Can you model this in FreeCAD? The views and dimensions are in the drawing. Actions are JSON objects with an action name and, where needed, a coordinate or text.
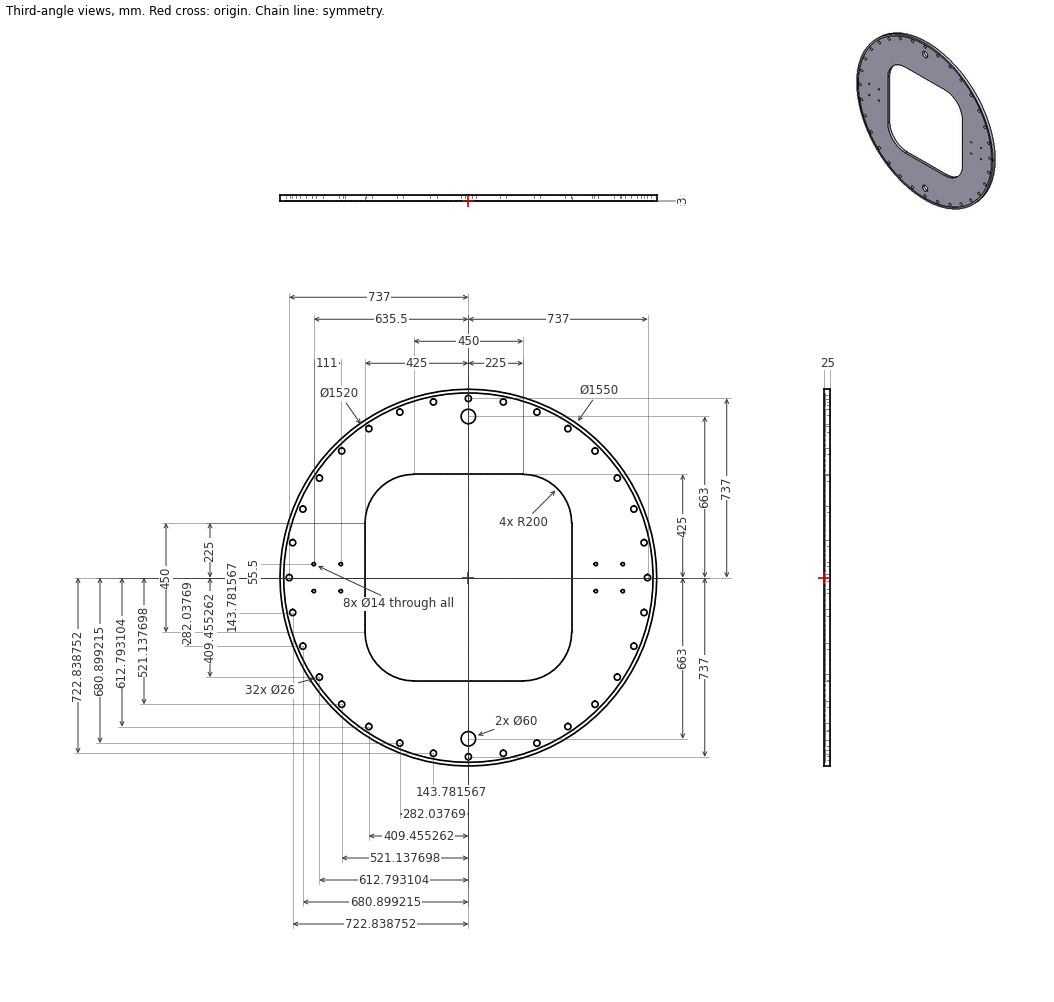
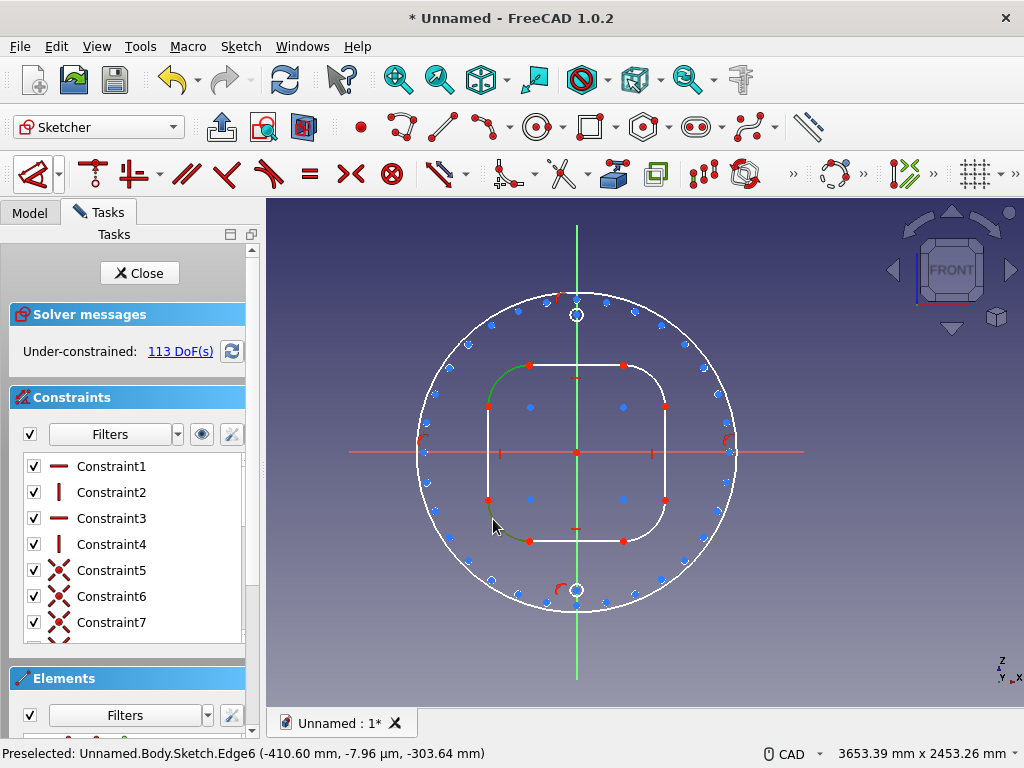
{"action": "left_click", "coordinate": [642, 537]}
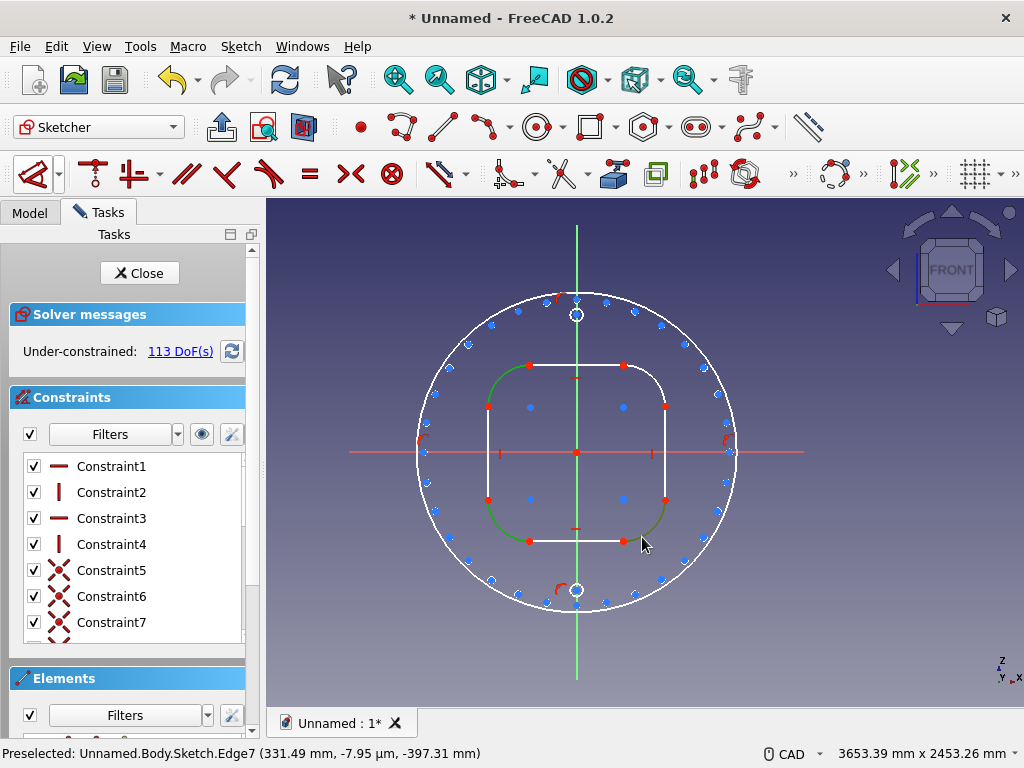
{"action": "left_click", "coordinate": [660, 388]}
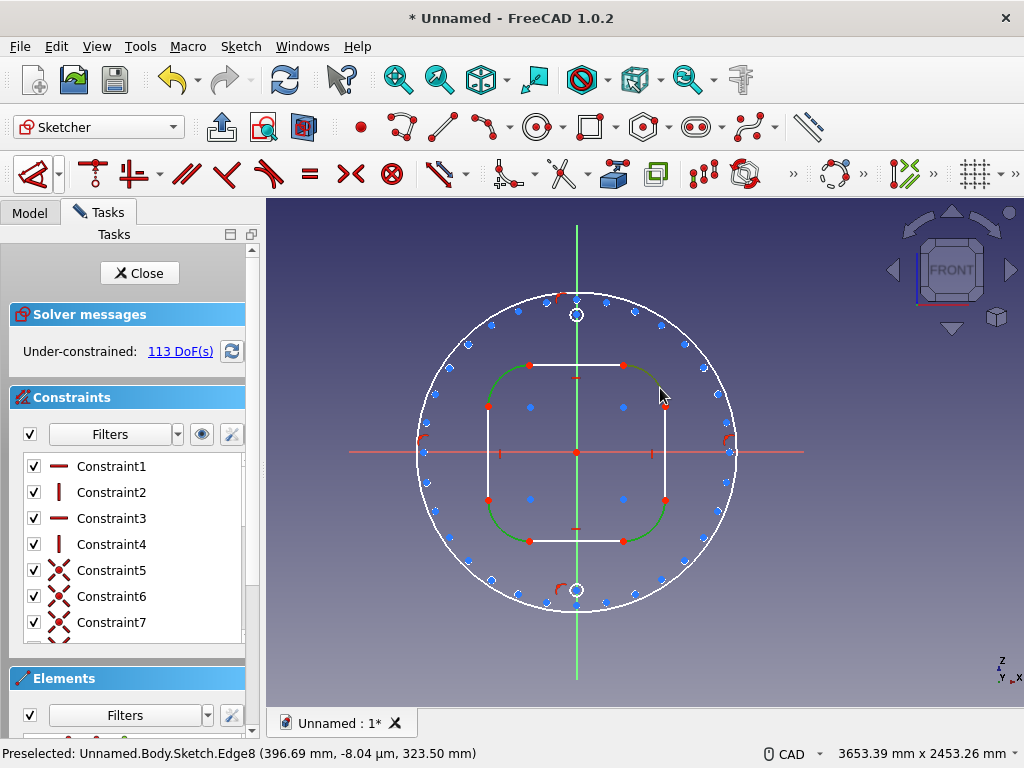
{"action": "left_click", "coordinate": [310, 174]}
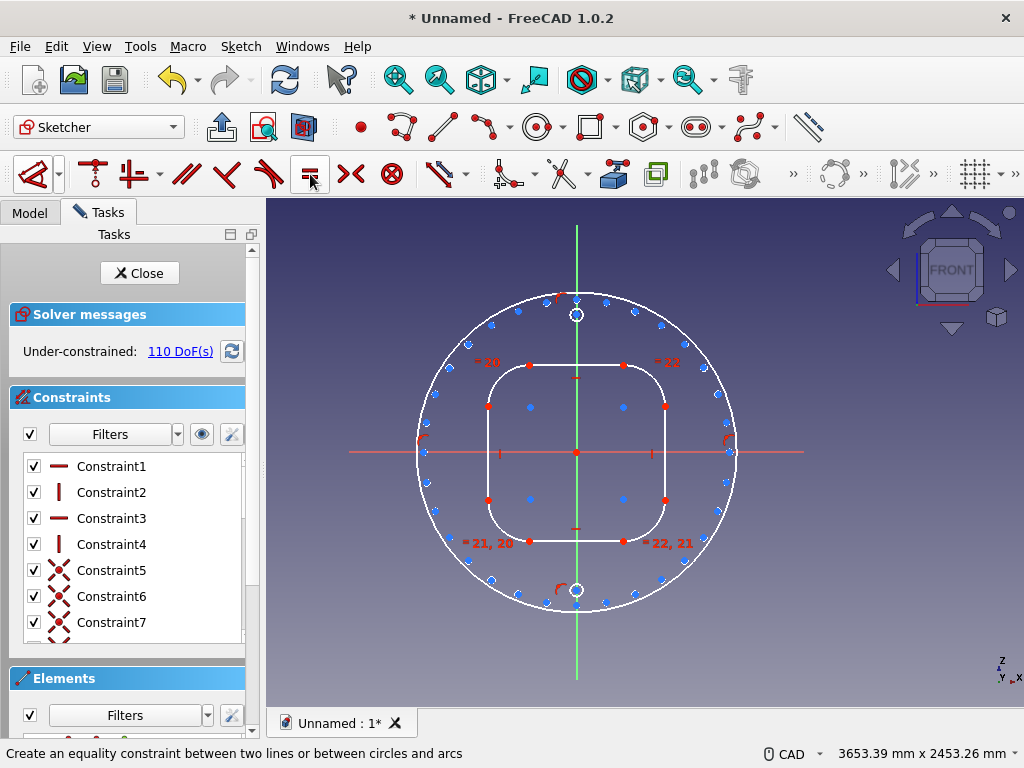
{"action": "scroll", "coordinate": [450, 535], "scroll_direction": "up", "scroll_amount": 9}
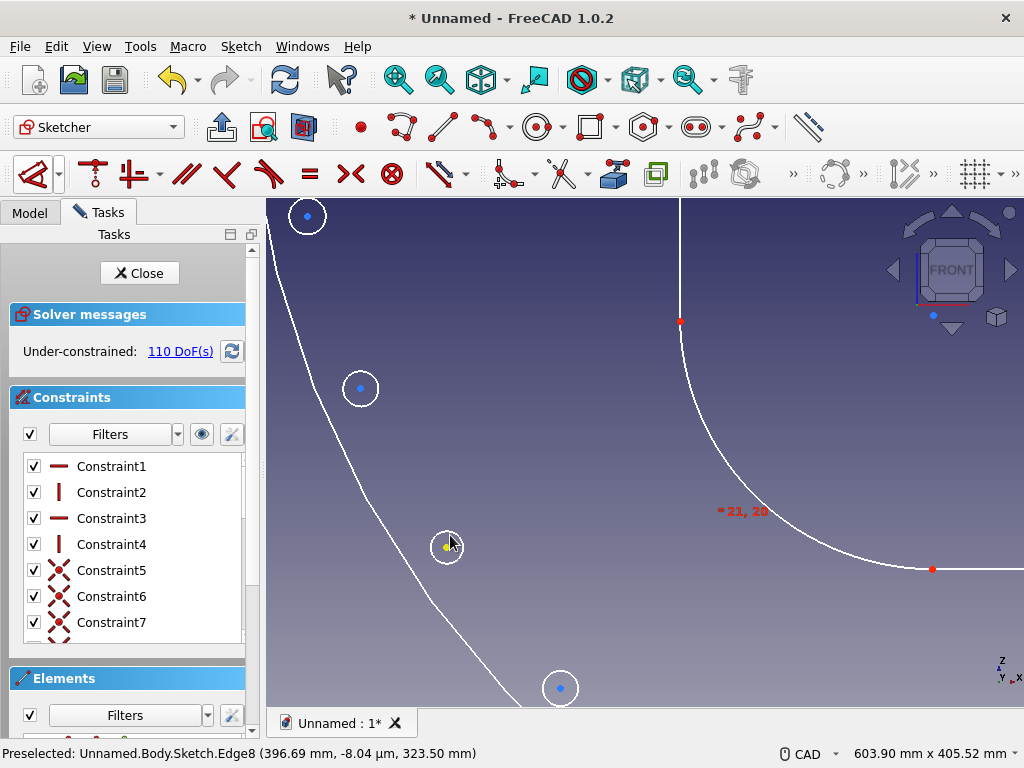
{"action": "left_click", "coordinate": [447, 531]}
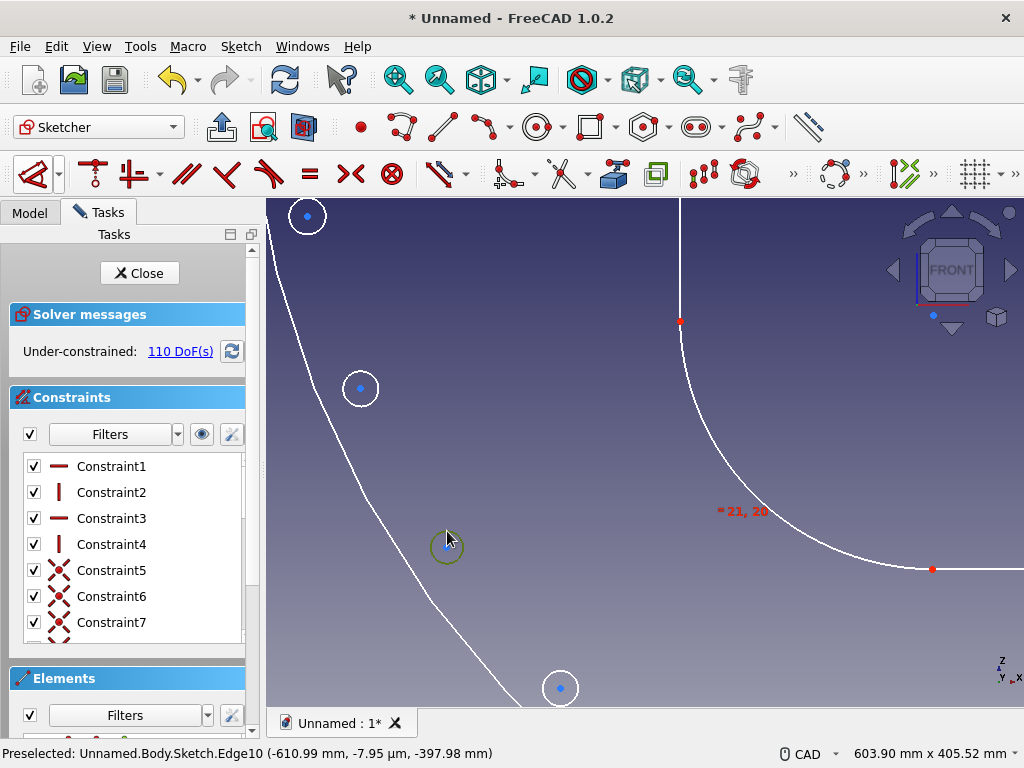
{"action": "scroll", "coordinate": [450, 536], "scroll_direction": "down", "scroll_amount": 9}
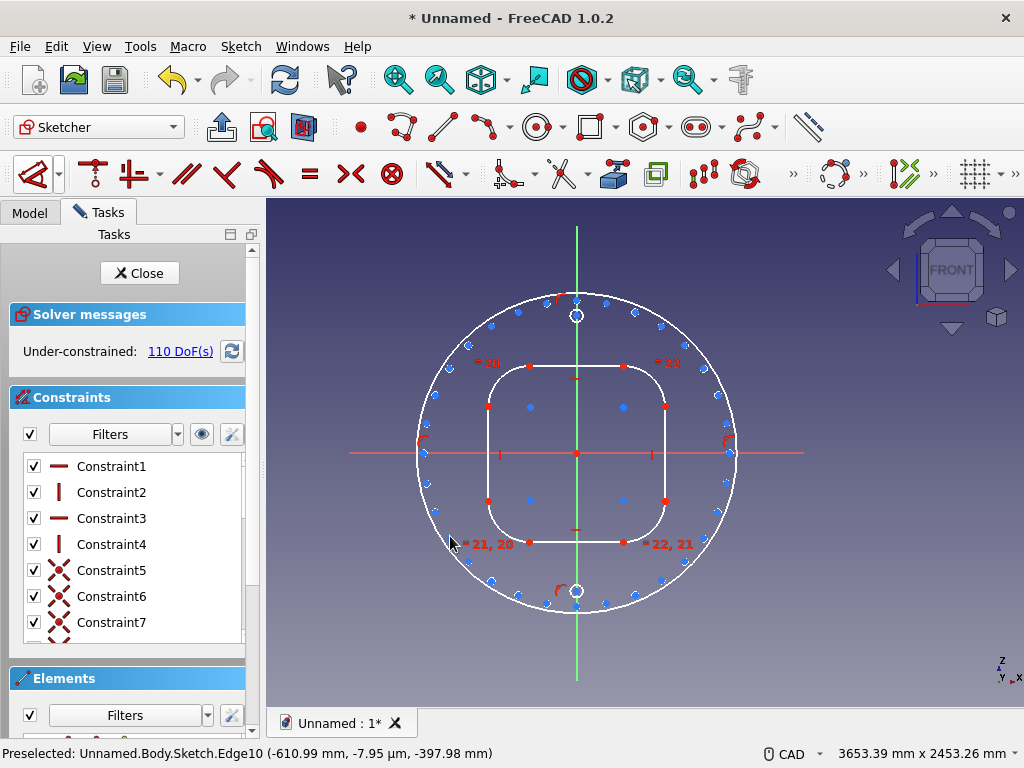
{"action": "scroll", "coordinate": [494, 579], "scroll_direction": "up", "scroll_amount": 8}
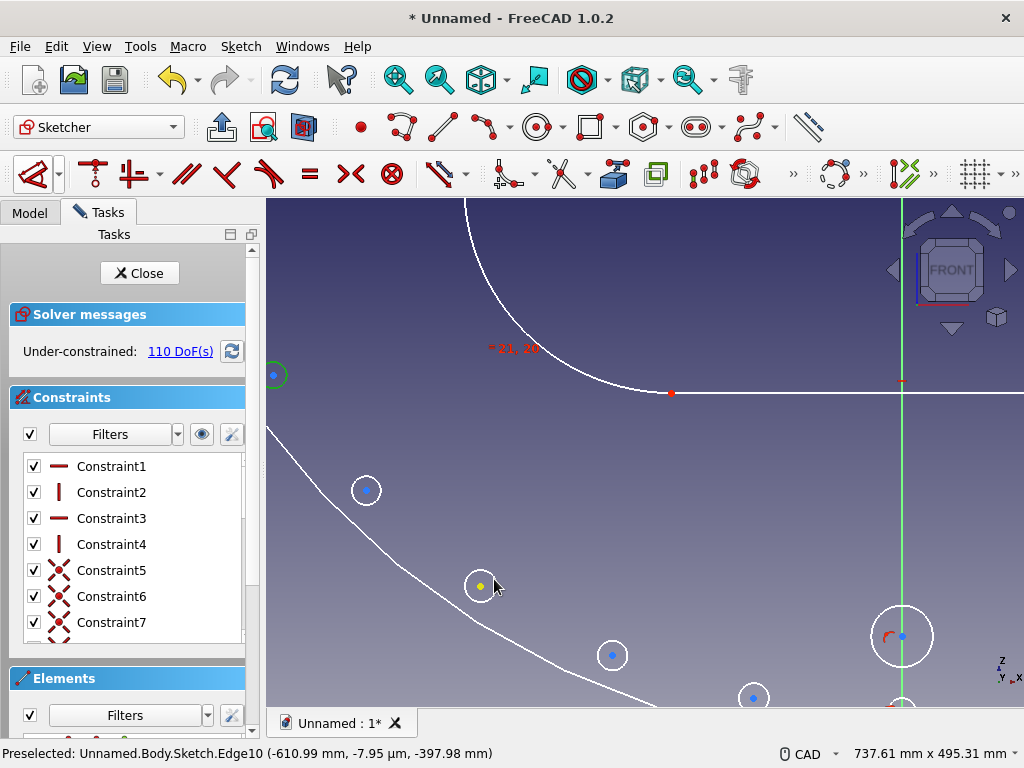
{"action": "left_click", "coordinate": [492, 575]}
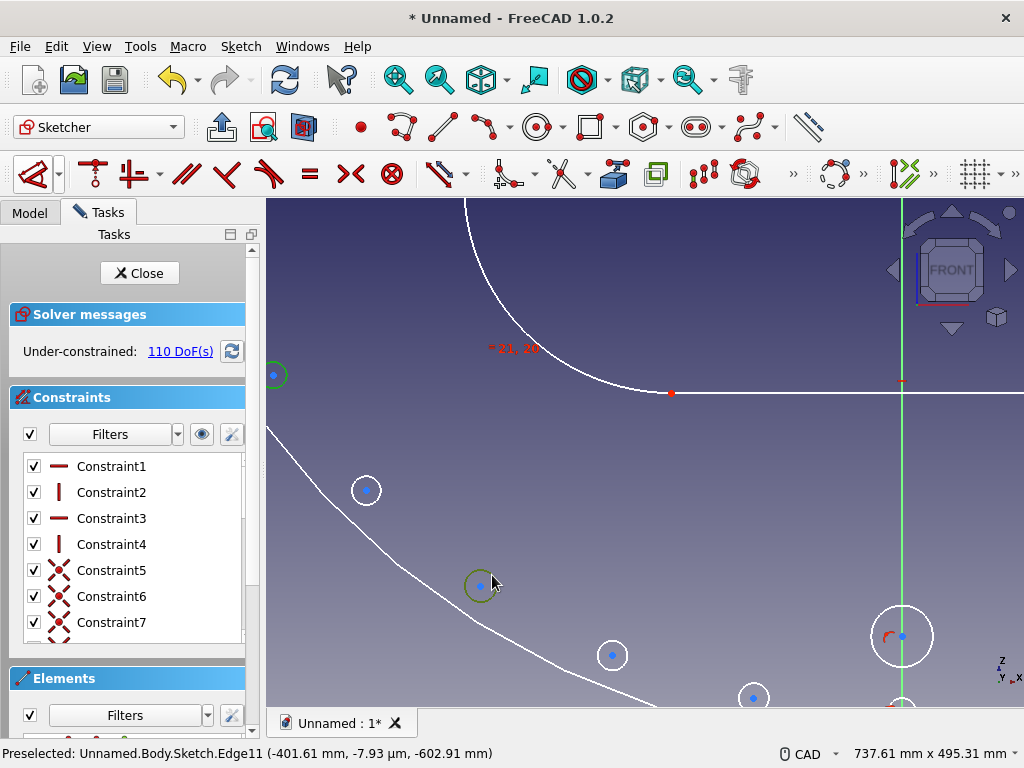
{"action": "left_click", "coordinate": [376, 480]}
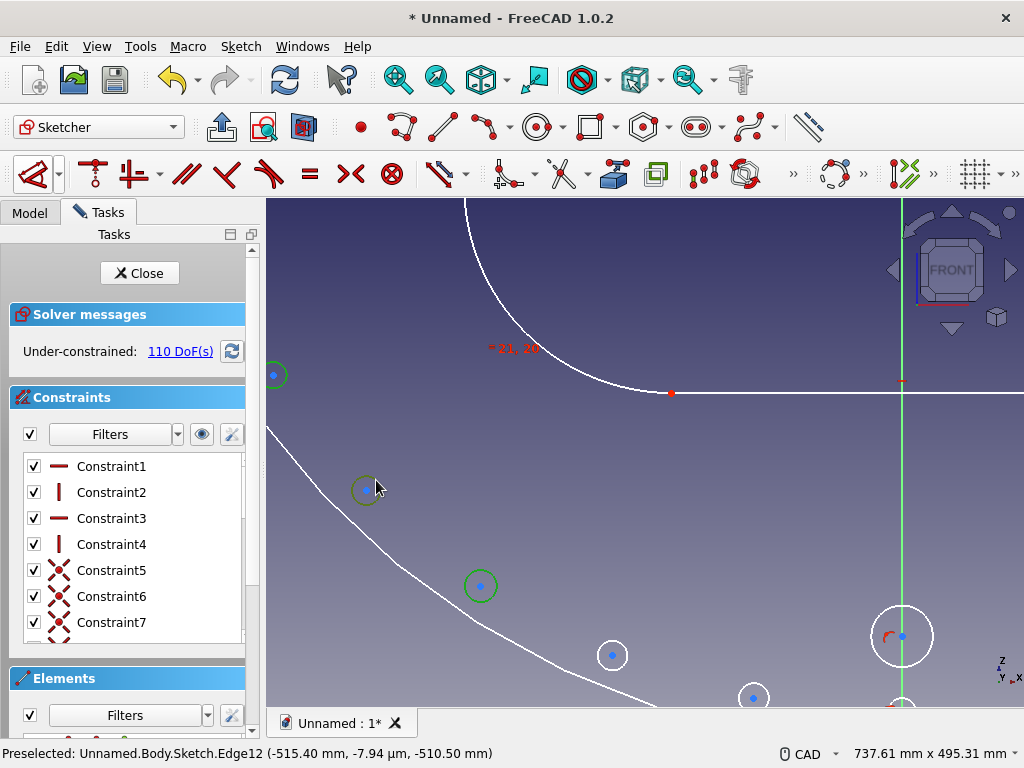
{"action": "scroll", "coordinate": [494, 579], "scroll_direction": "down", "scroll_amount": 8}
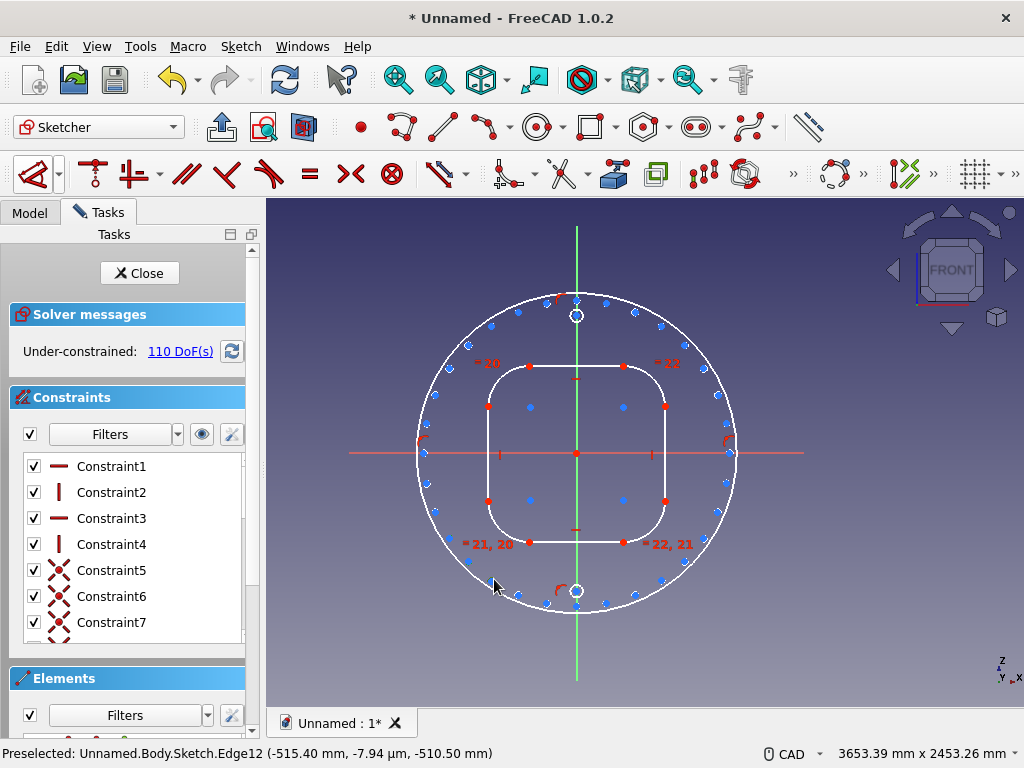
{"action": "scroll", "coordinate": [438, 510], "scroll_direction": "up", "scroll_amount": 8}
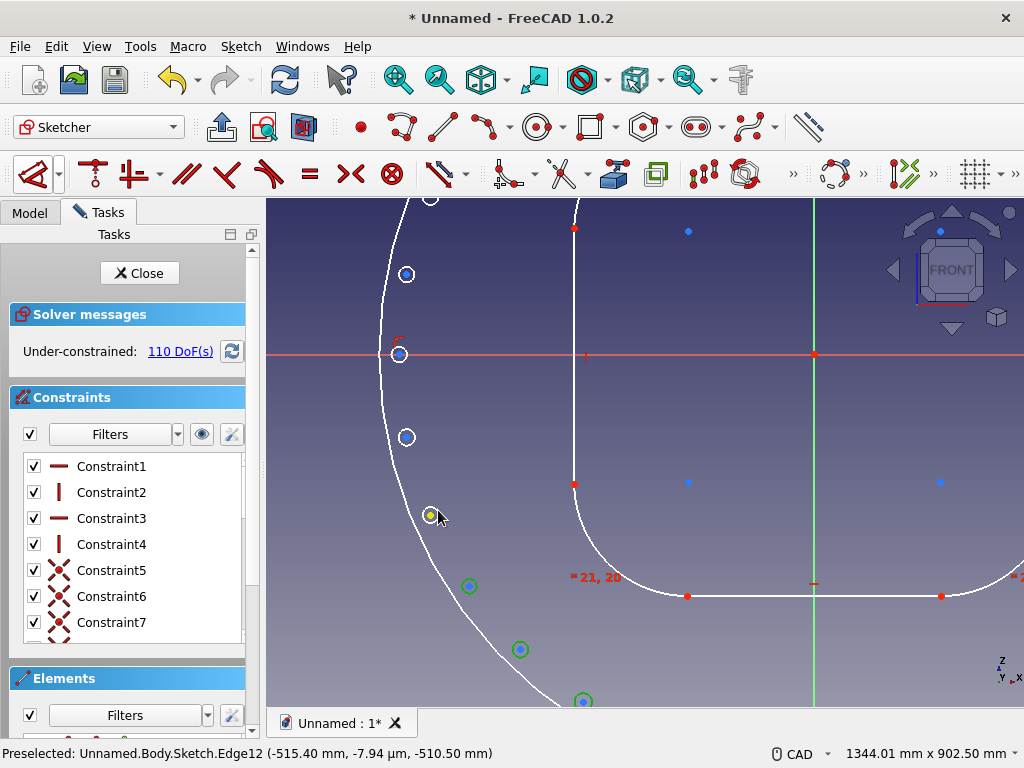
{"action": "left_click", "coordinate": [435, 508]}